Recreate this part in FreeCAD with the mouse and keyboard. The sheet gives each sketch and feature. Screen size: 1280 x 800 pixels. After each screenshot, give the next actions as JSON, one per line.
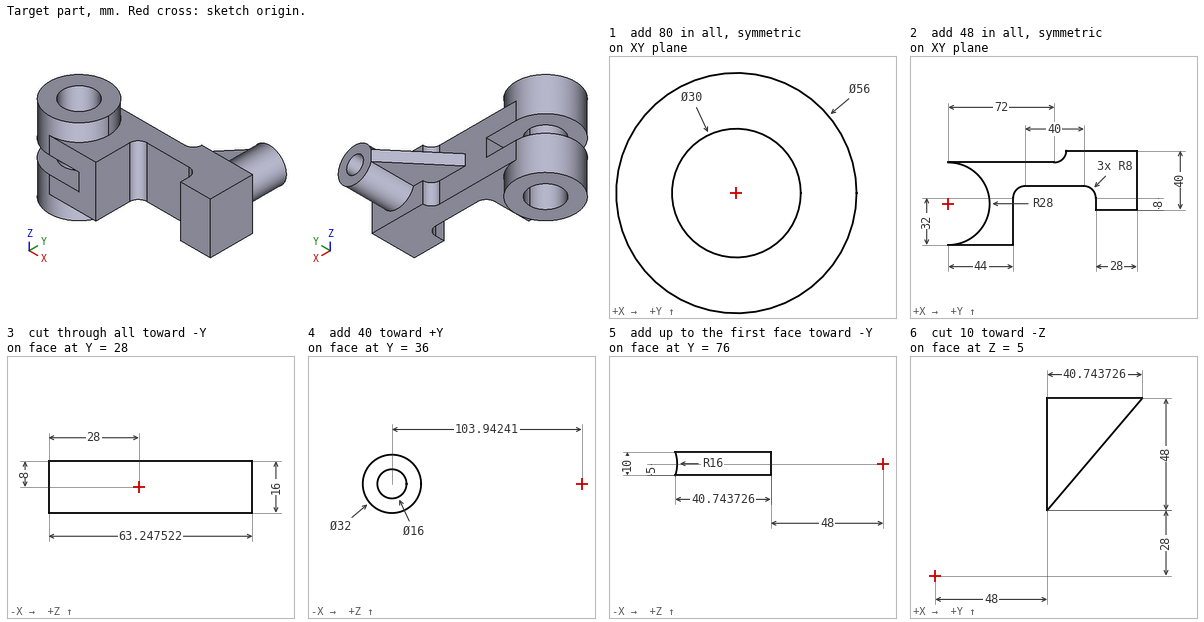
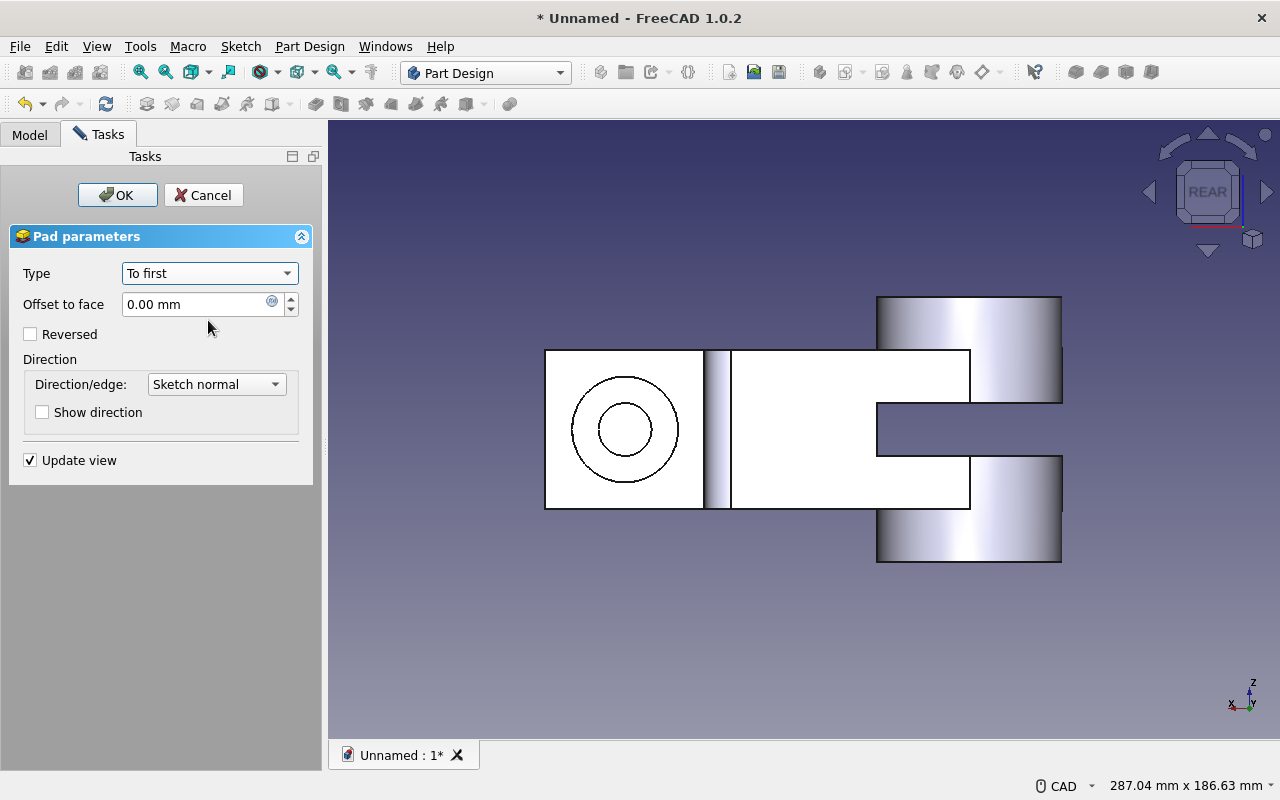
{"action": "left_click", "coordinate": [31, 334]}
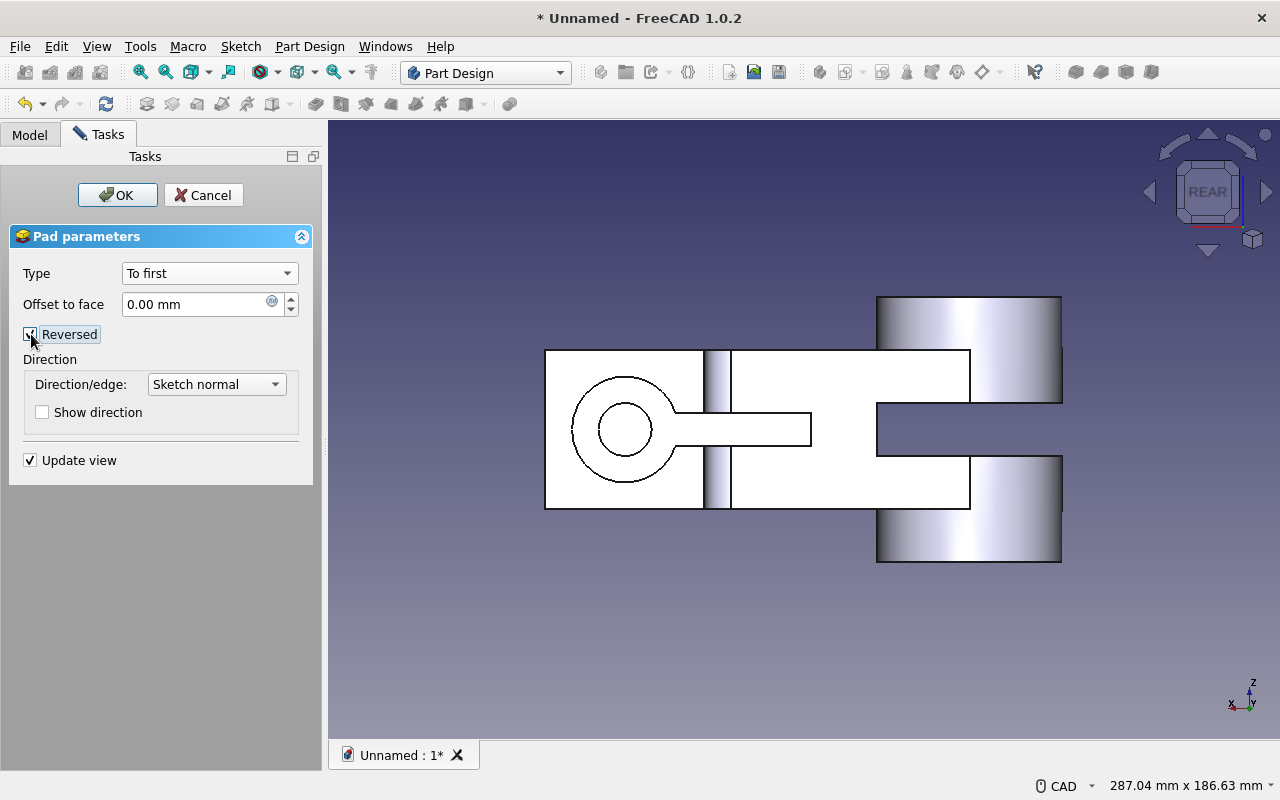
{"action": "left_click", "coordinate": [118, 195]}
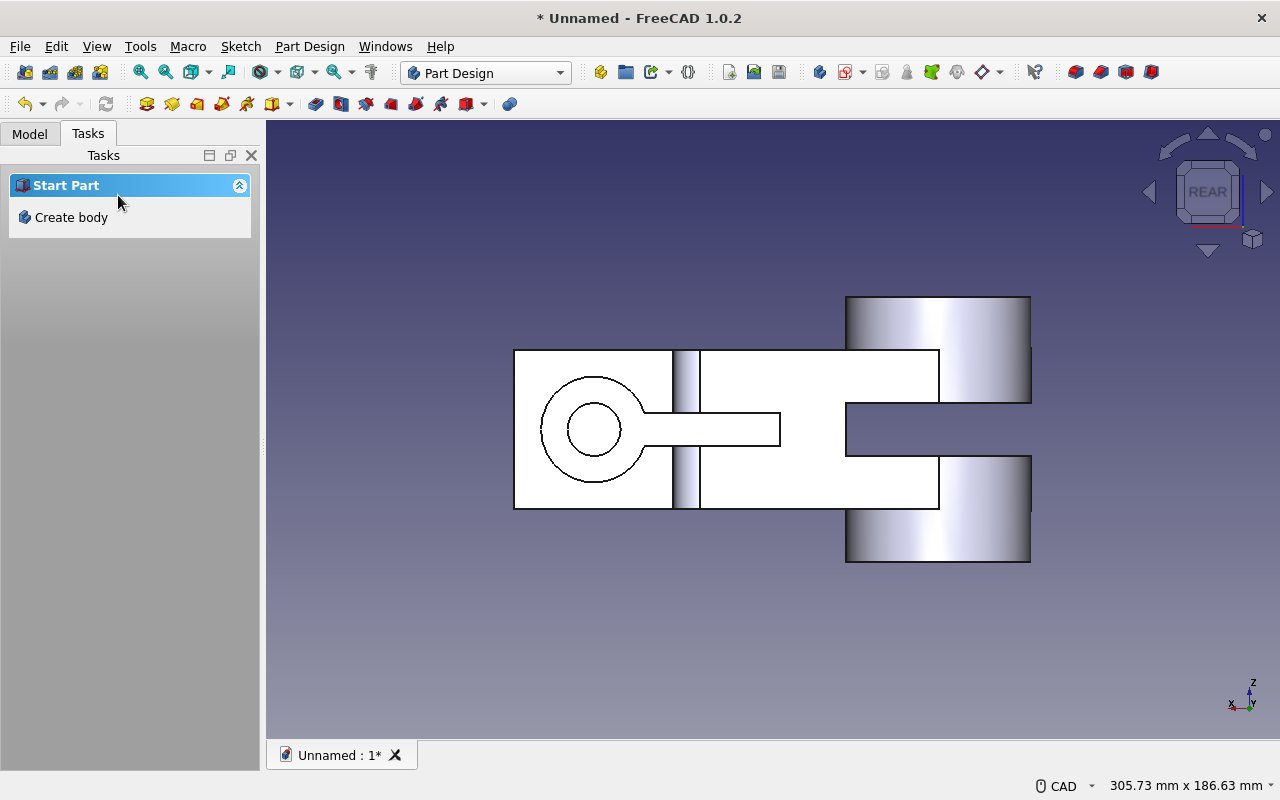
{"action": "key", "text": "0"}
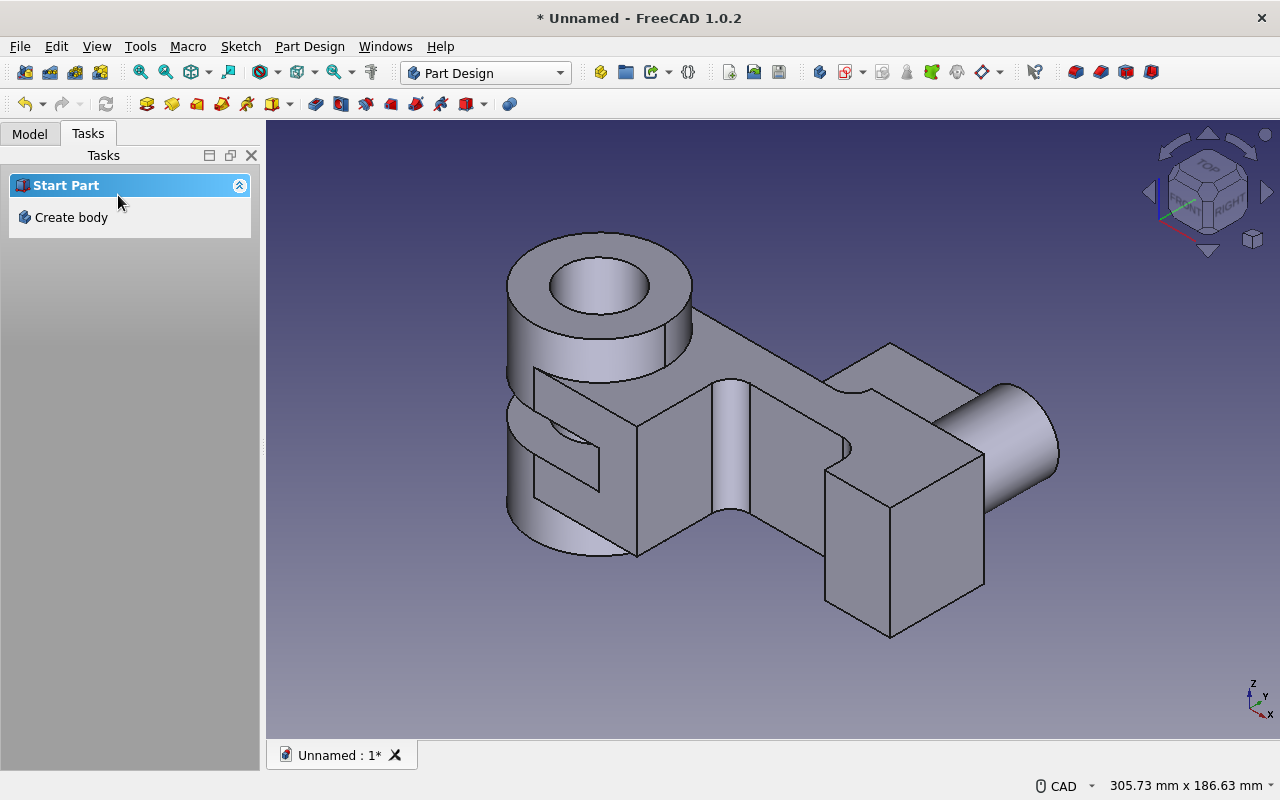
{"action": "key", "text": "2"}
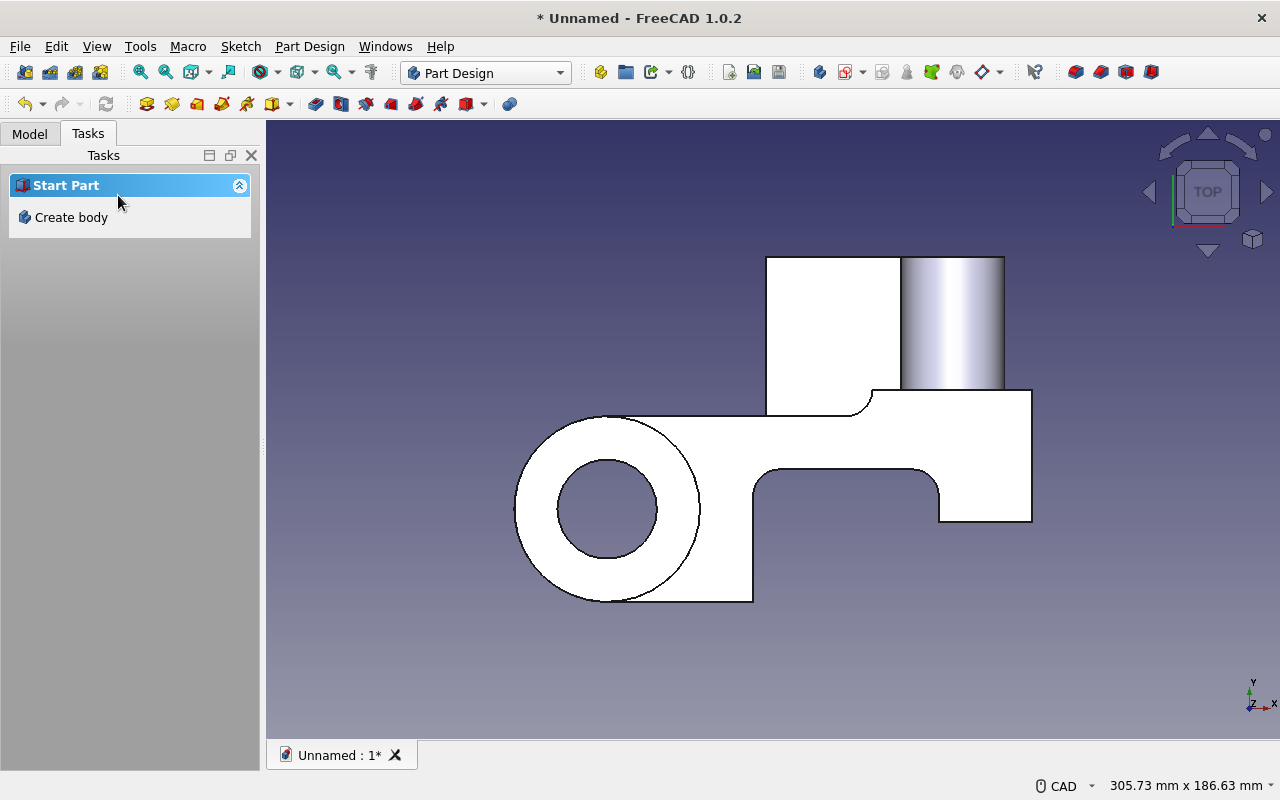
{"action": "left_click", "coordinate": [834, 336]}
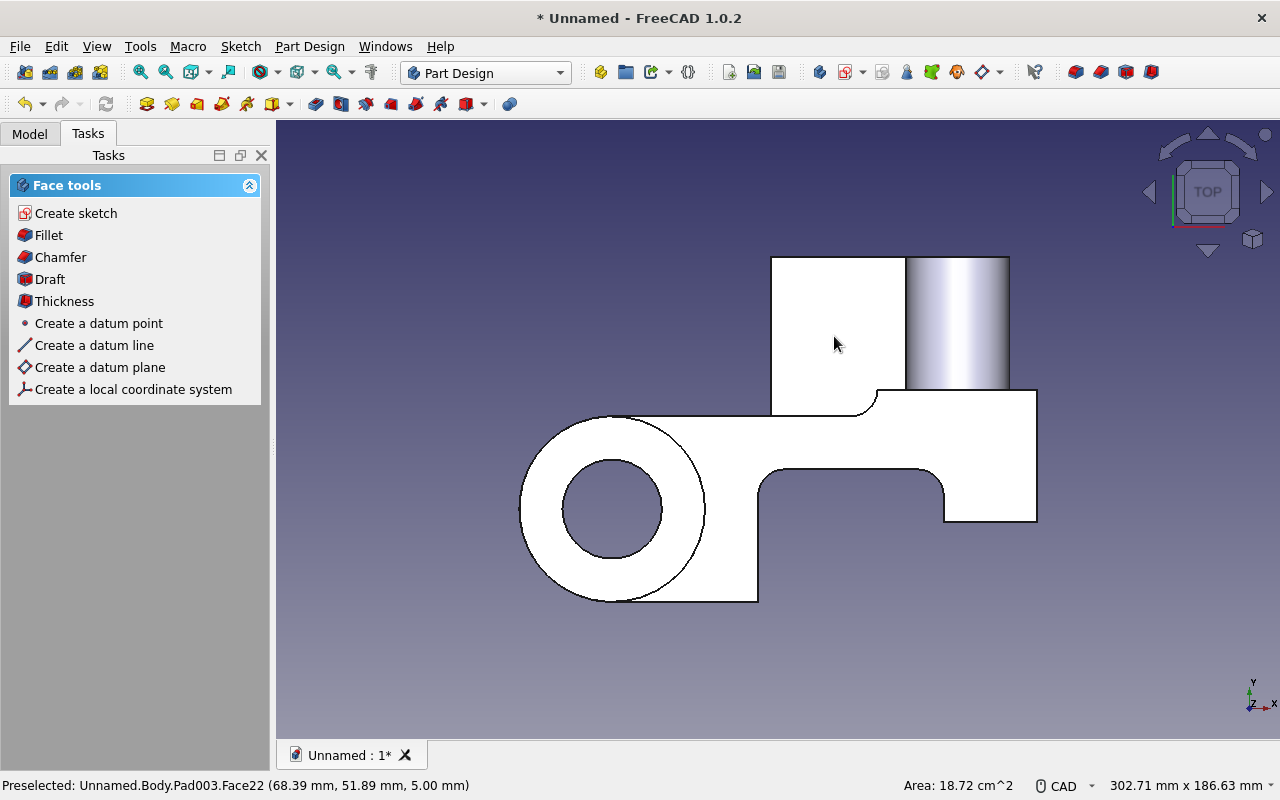
{"action": "left_click", "coordinate": [844, 72]}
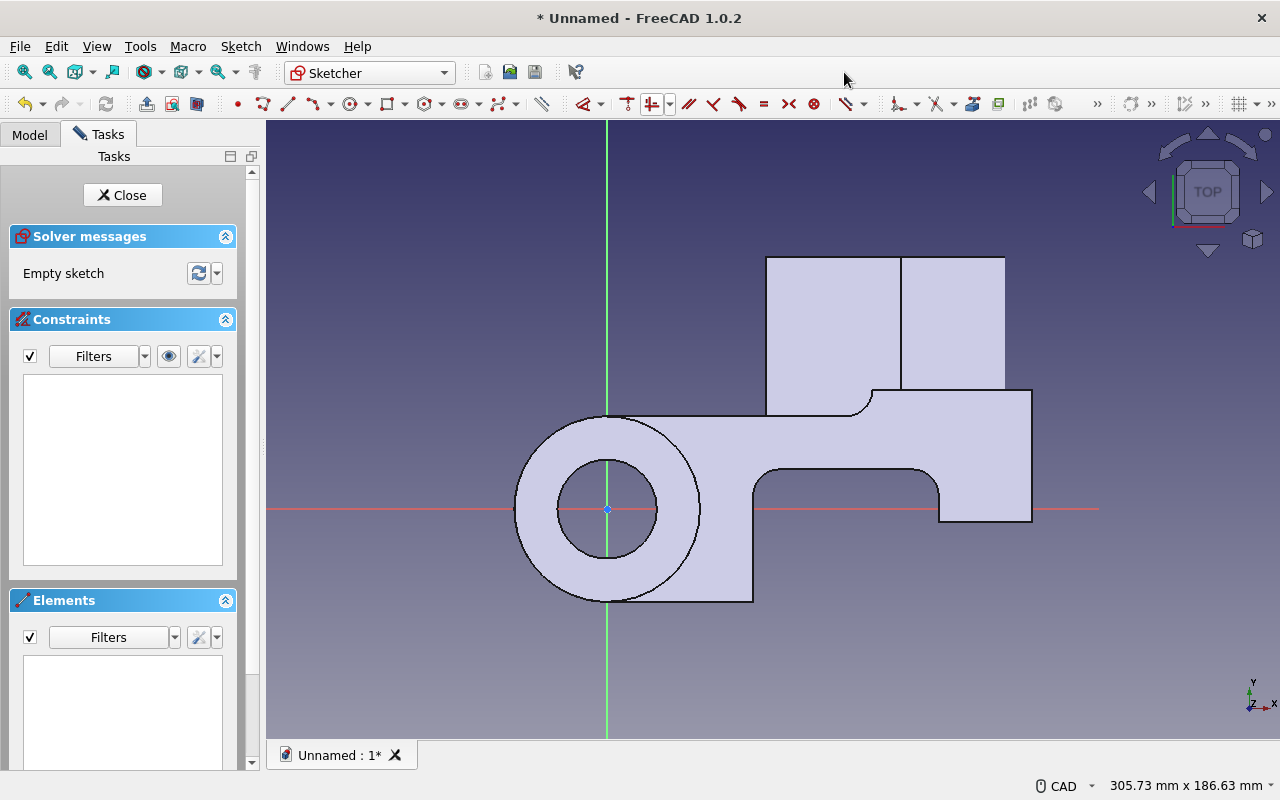
{"action": "left_click", "coordinate": [197, 104]}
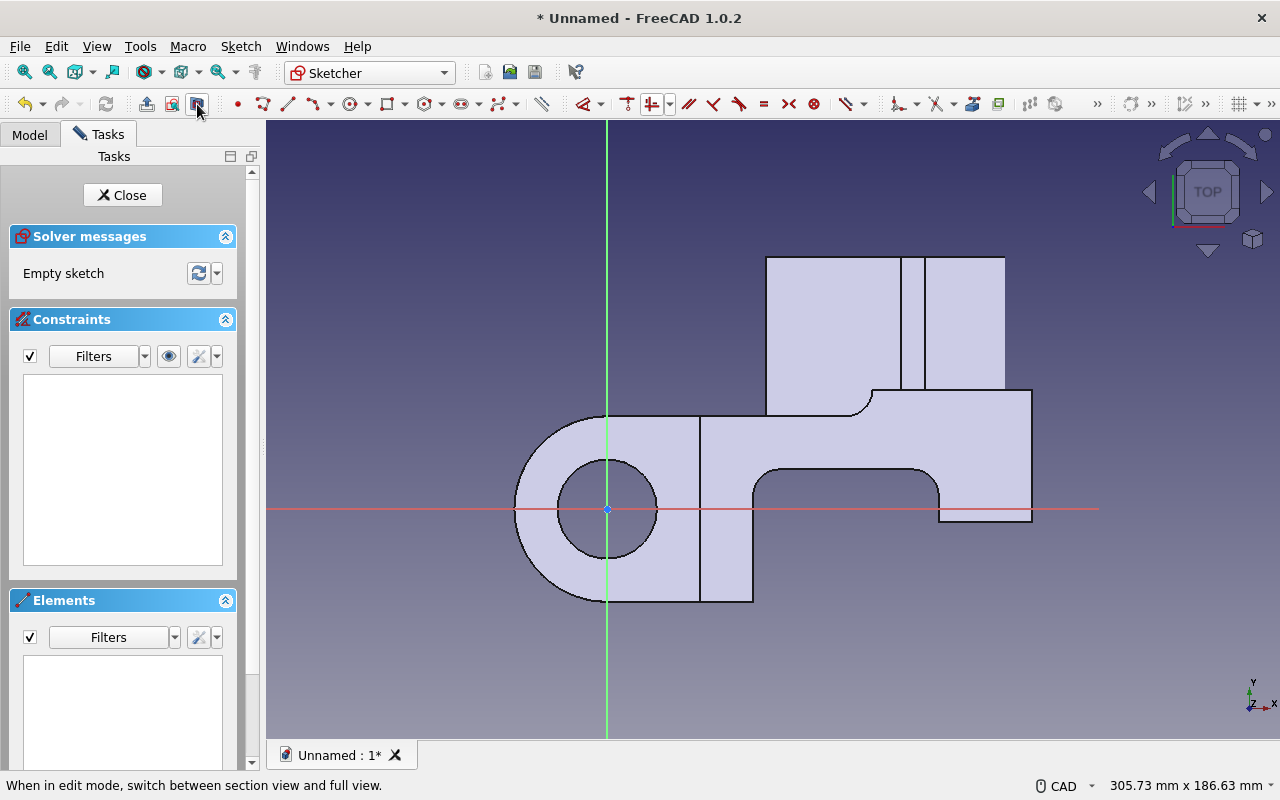
{"action": "scroll", "coordinate": [856, 289], "scroll_direction": "up", "scroll_amount": 2}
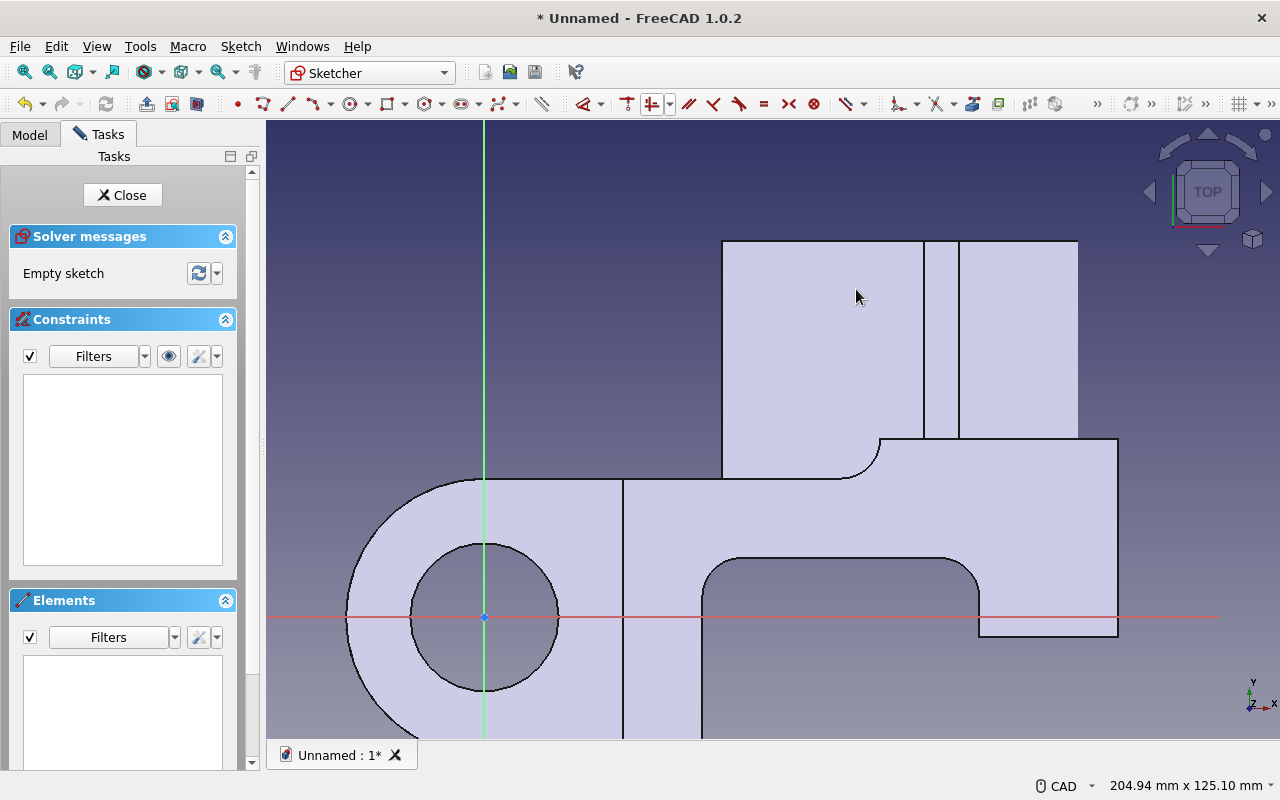
{"action": "left_click", "coordinate": [263, 104]}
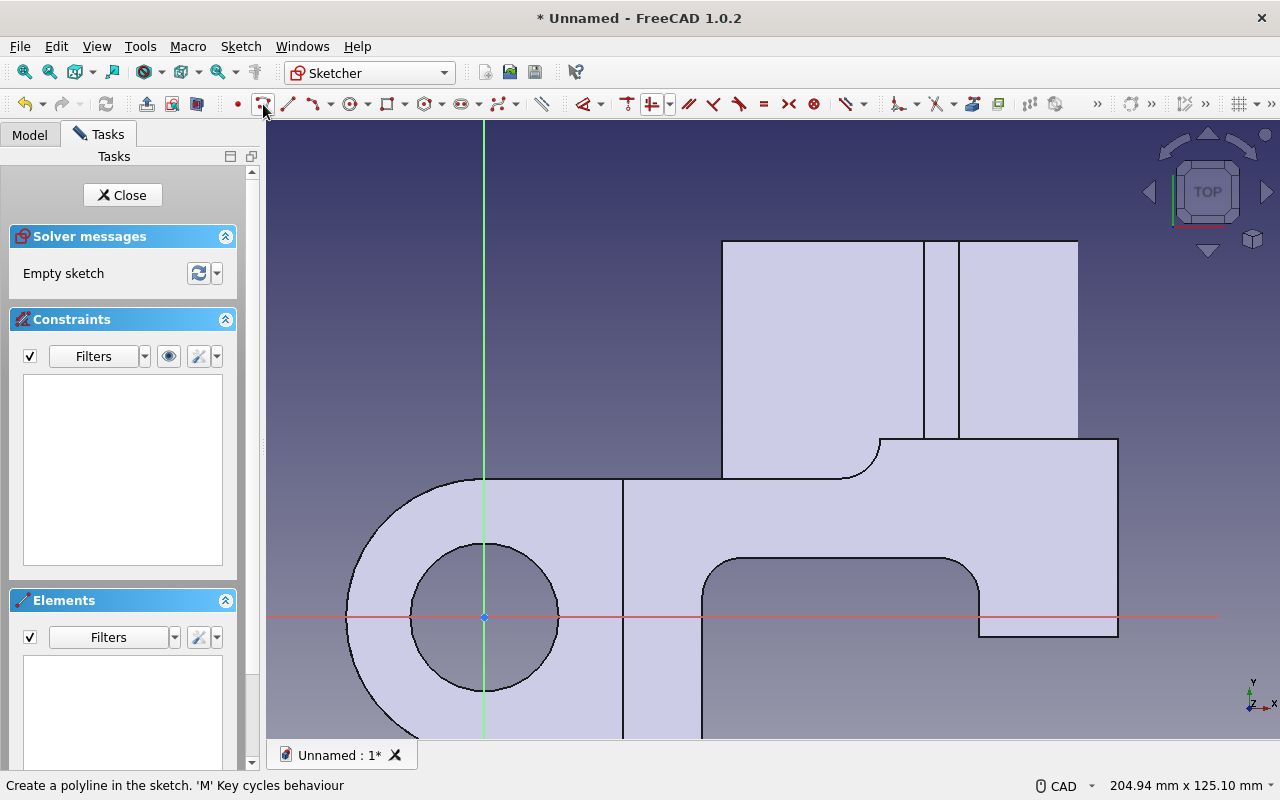
{"action": "left_click", "coordinate": [722, 479]}
{"action": "left_click", "coordinate": [924, 241]}
{"action": "left_click", "coordinate": [722, 241]}
{"action": "left_click", "coordinate": [722, 480]}
{"action": "key", "text": "Escape"}
{"action": "key", "text": "Escape"}